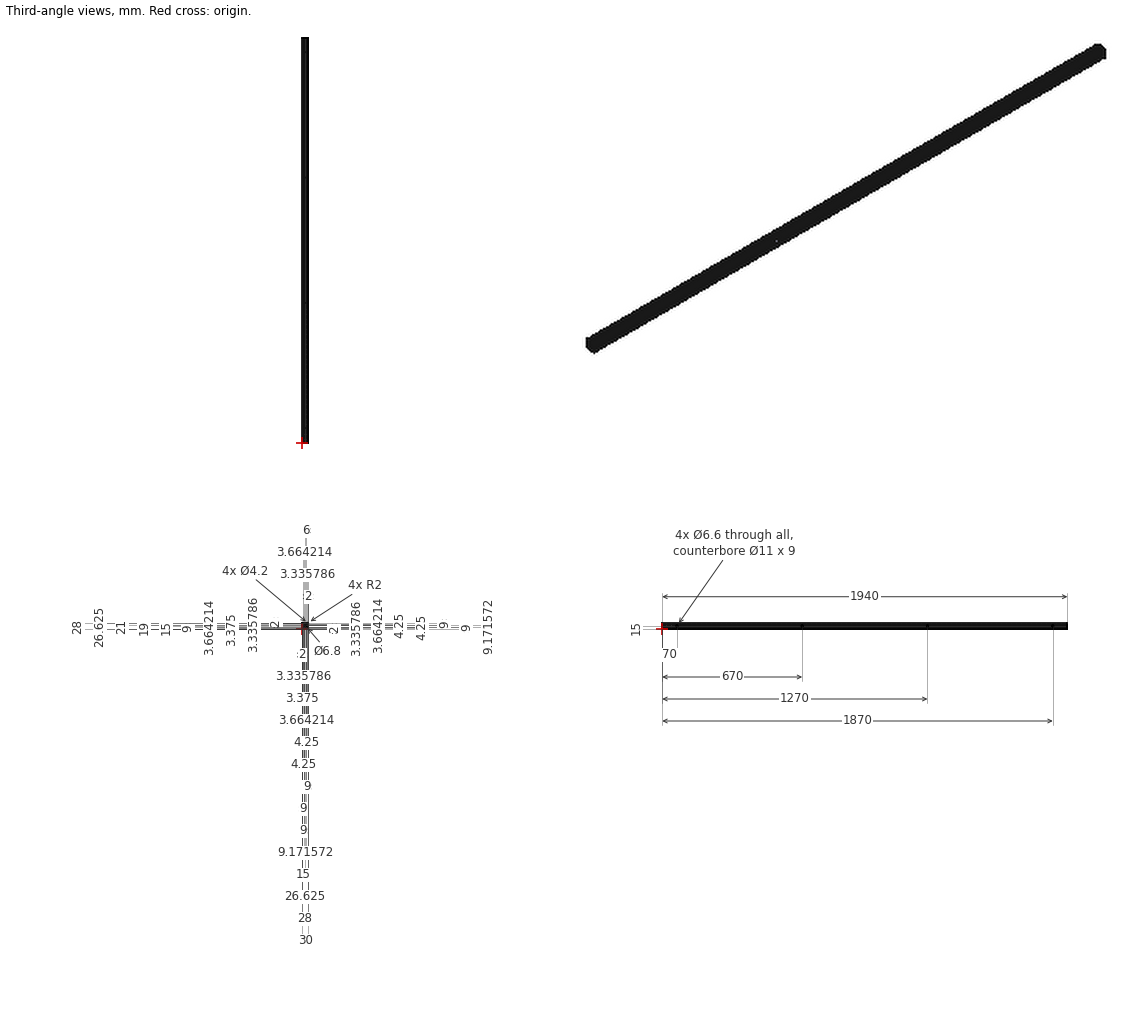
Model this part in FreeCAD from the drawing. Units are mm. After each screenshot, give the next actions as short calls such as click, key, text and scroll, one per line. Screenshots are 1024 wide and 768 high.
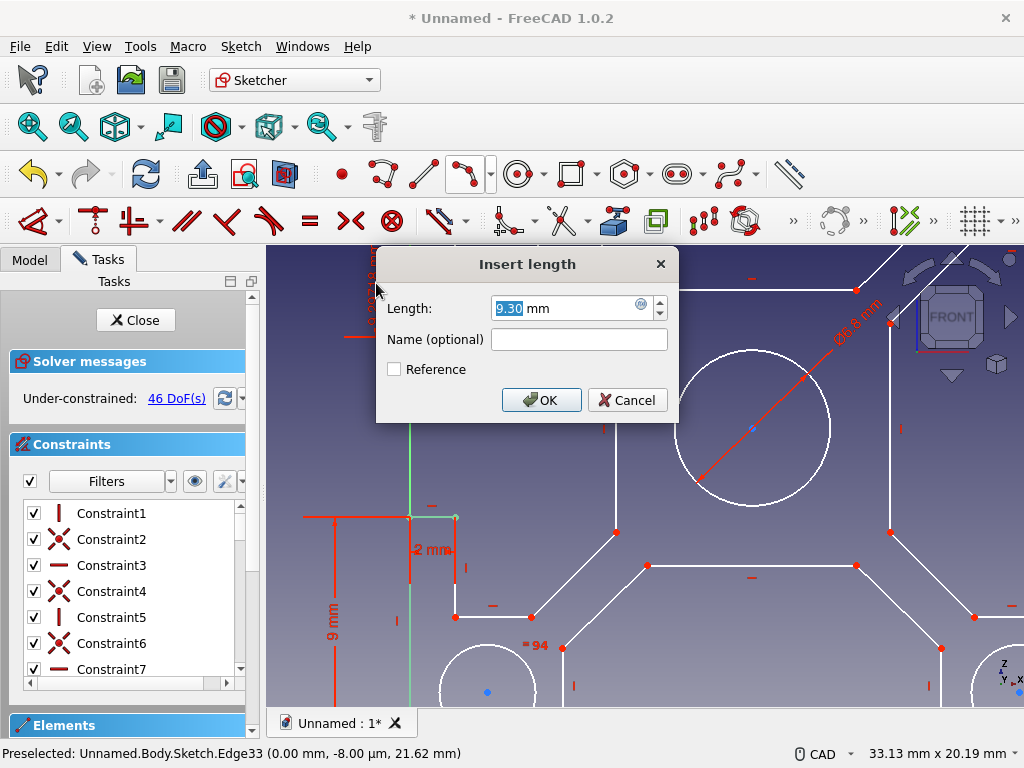
text(9)
key(Return)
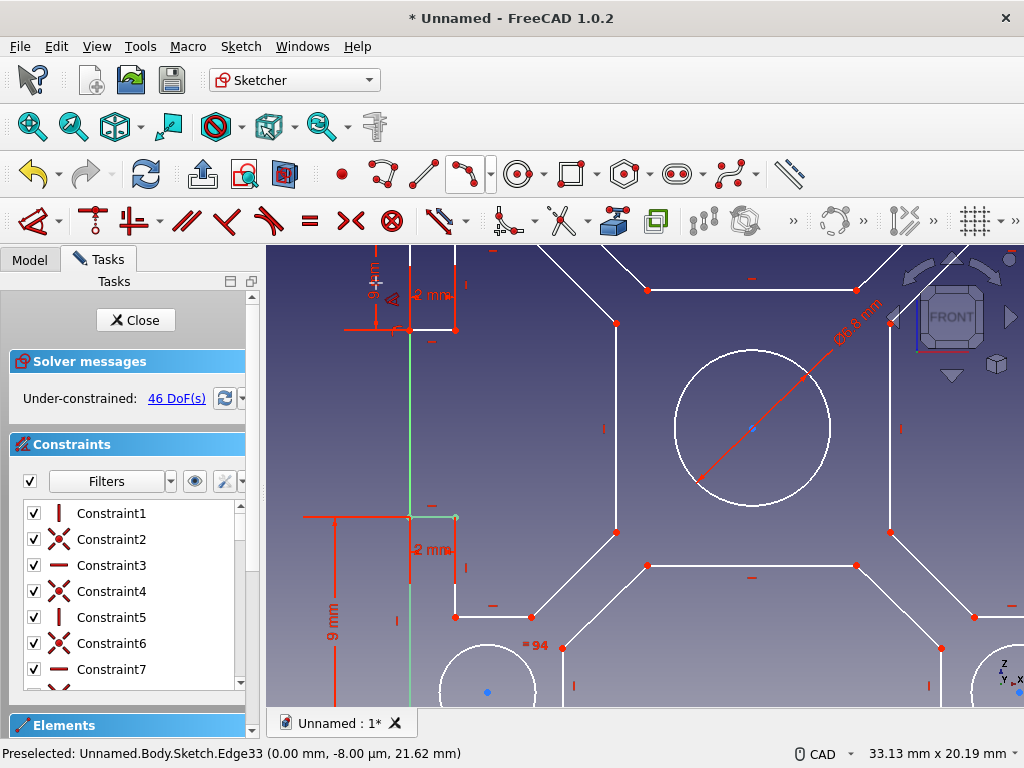
scroll(433, 517, down, 4)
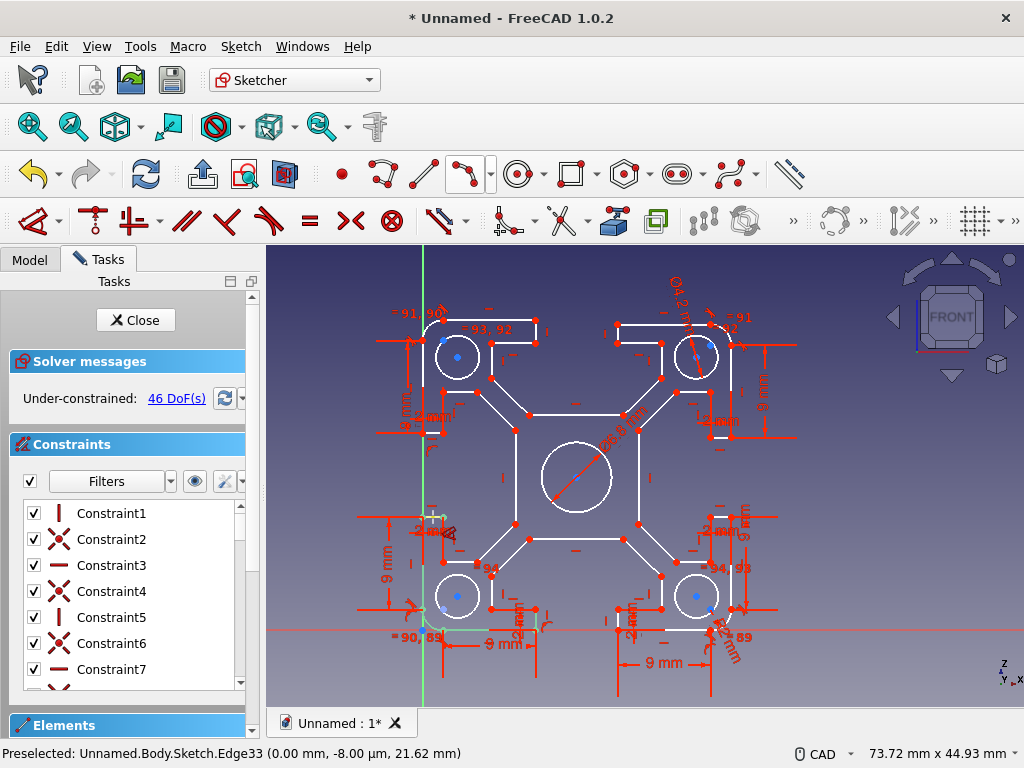
click(471, 320)
click(489, 286)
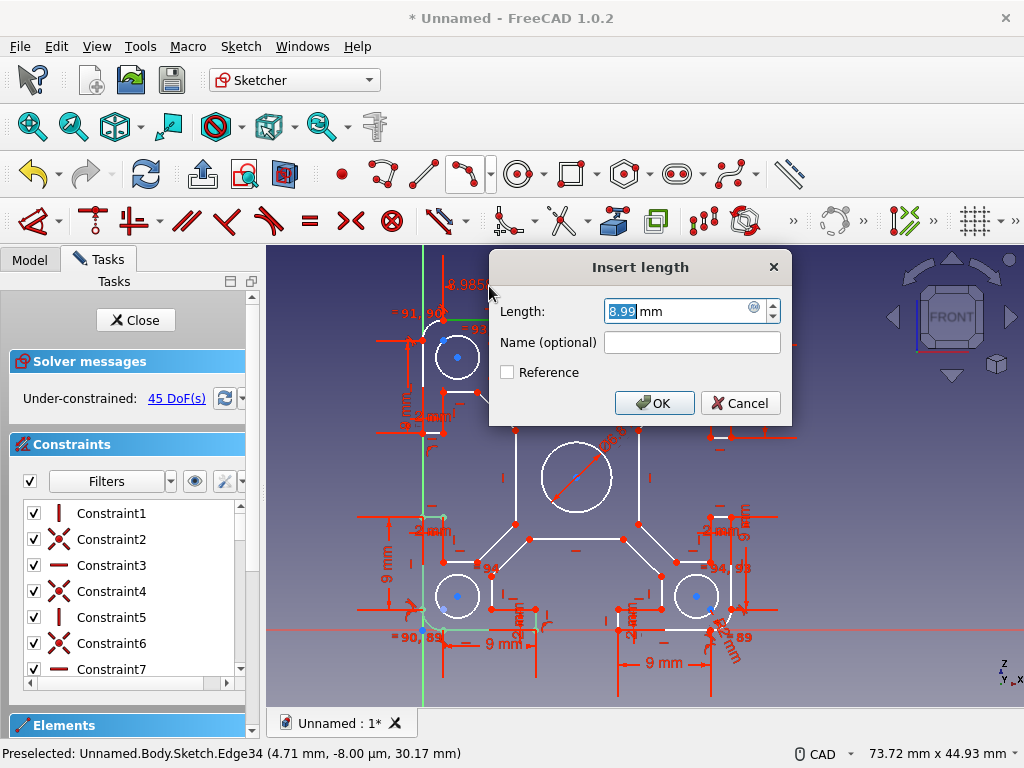
text(9)
key(Return)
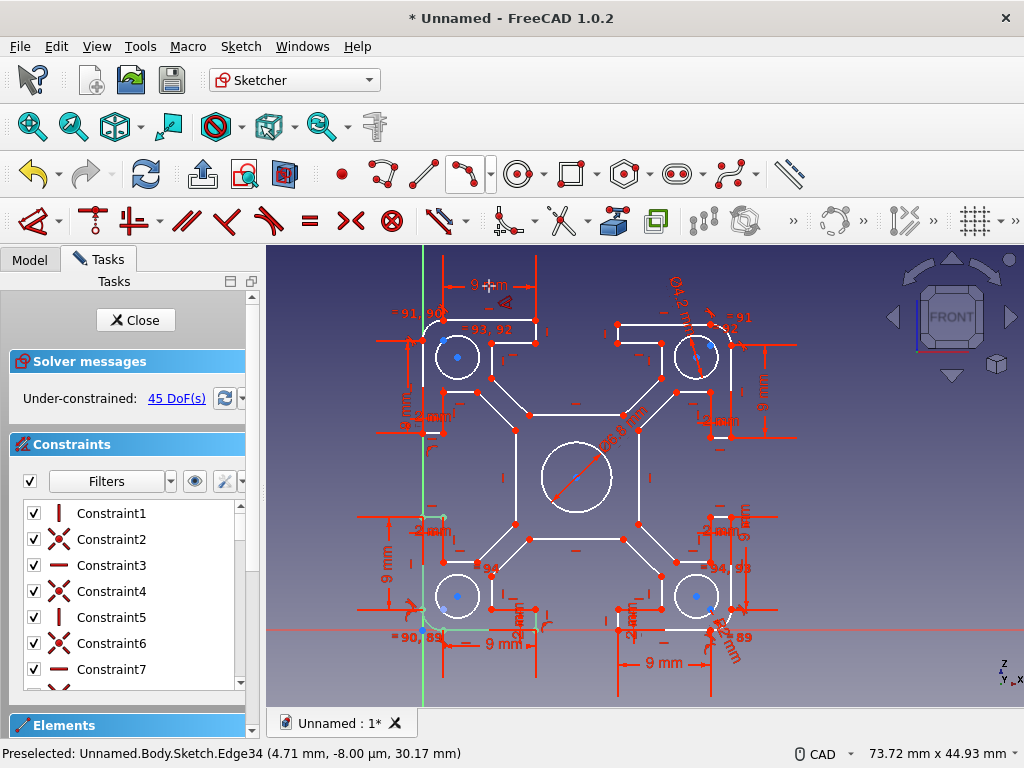
scroll(536, 329, up, 4)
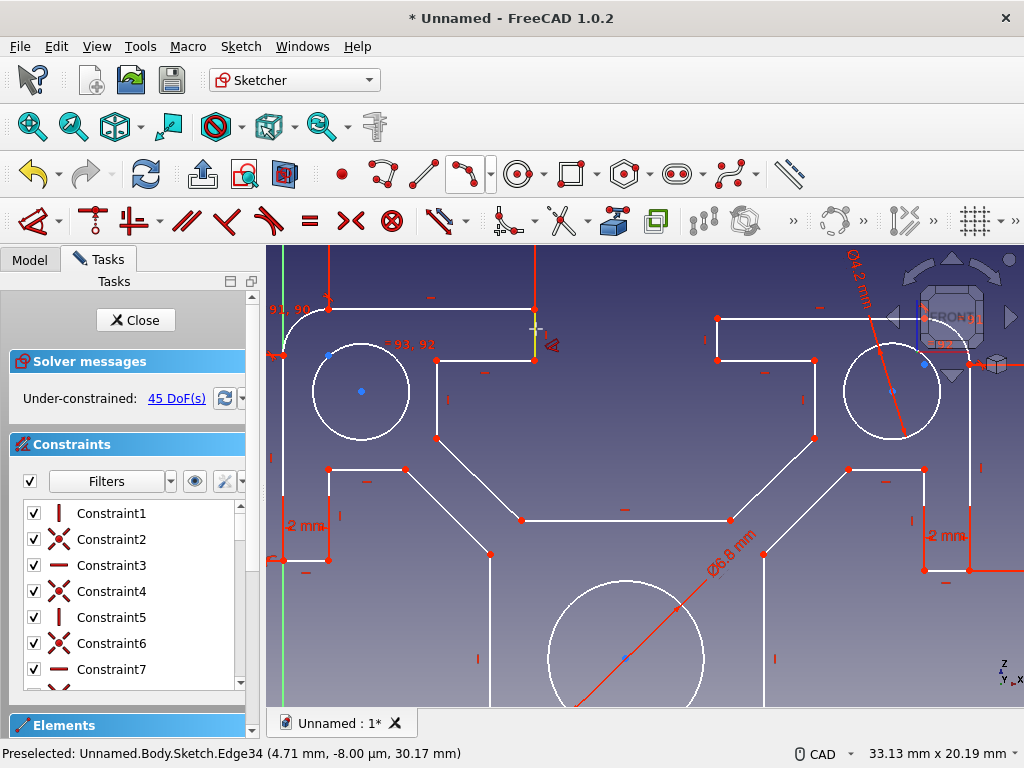
click(535, 330)
click(501, 335)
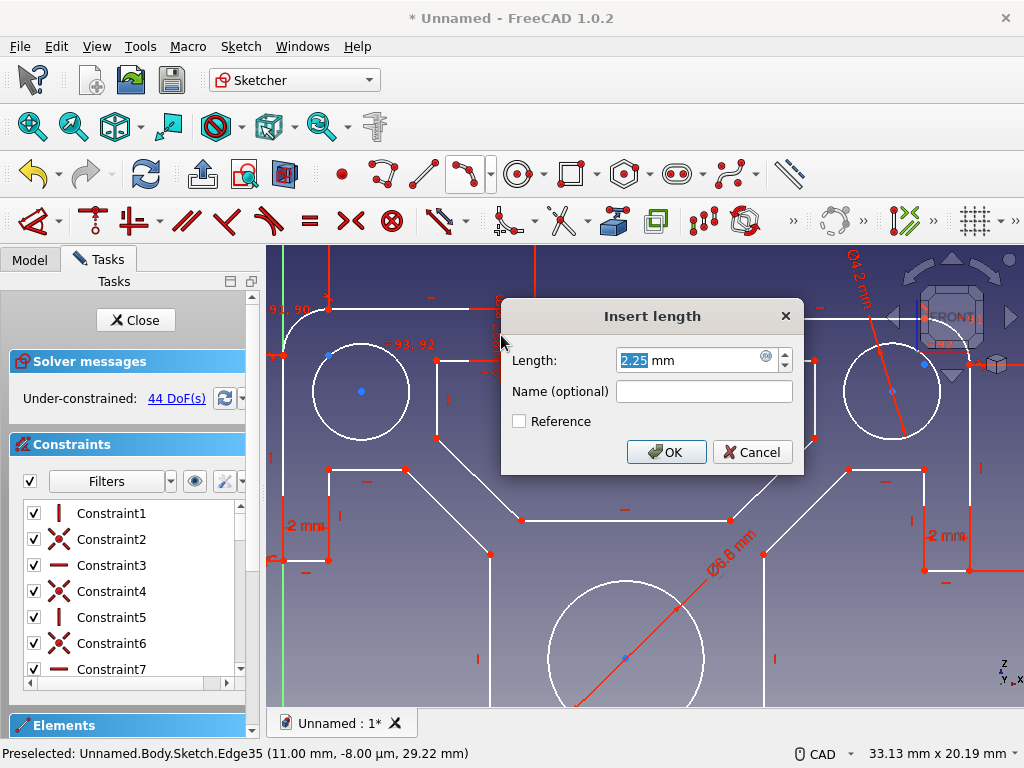
text(2)
key(Return)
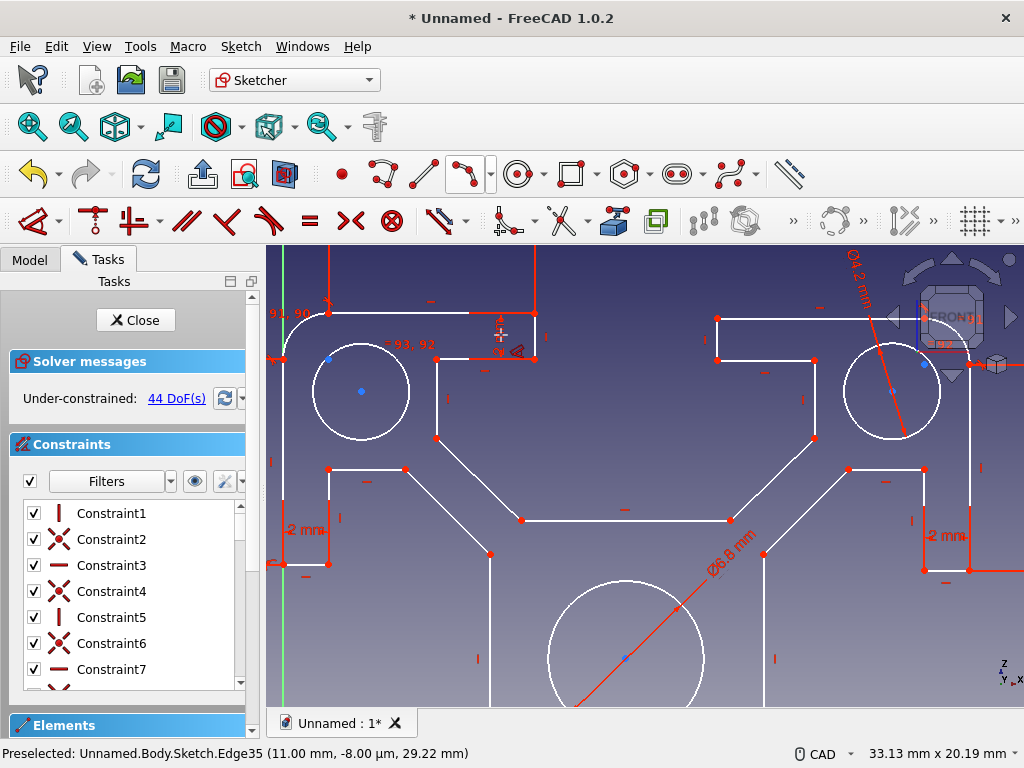
click(717, 348)
click(751, 340)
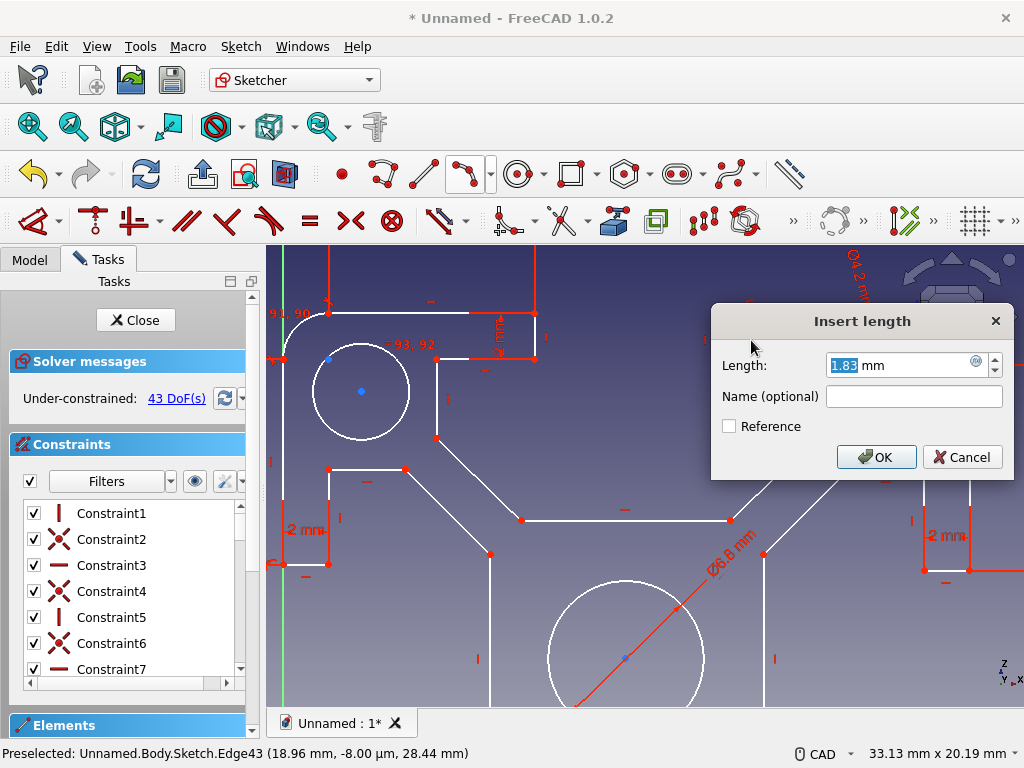
text(2)
key(Return)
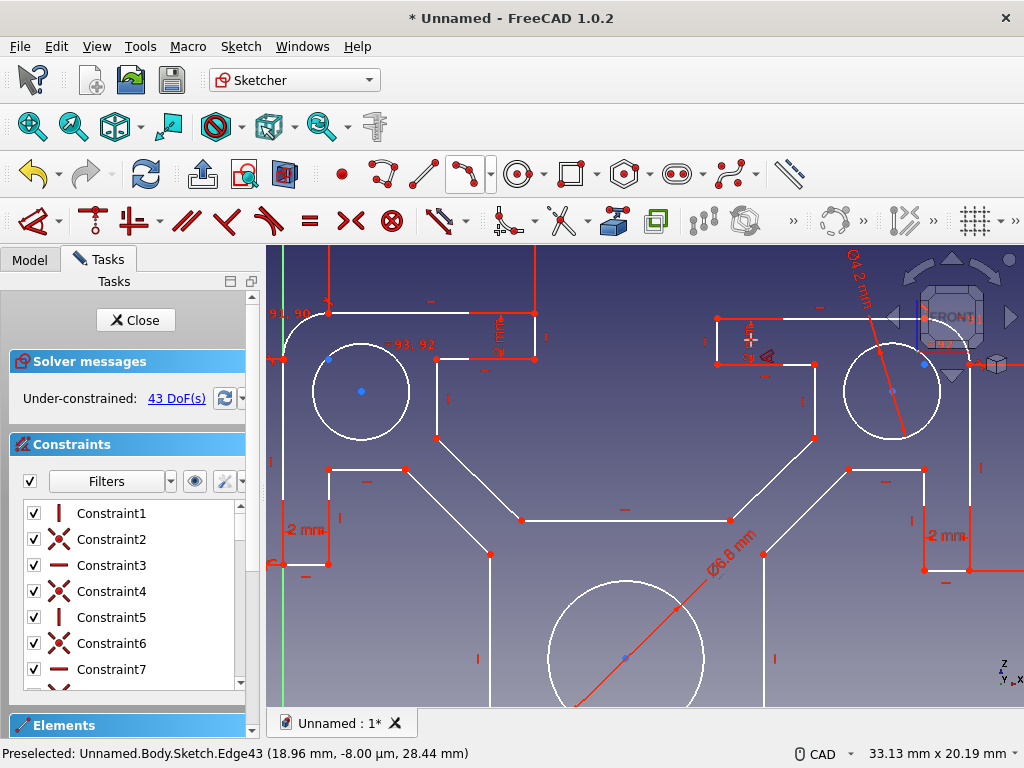
click(779, 319)
click(788, 285)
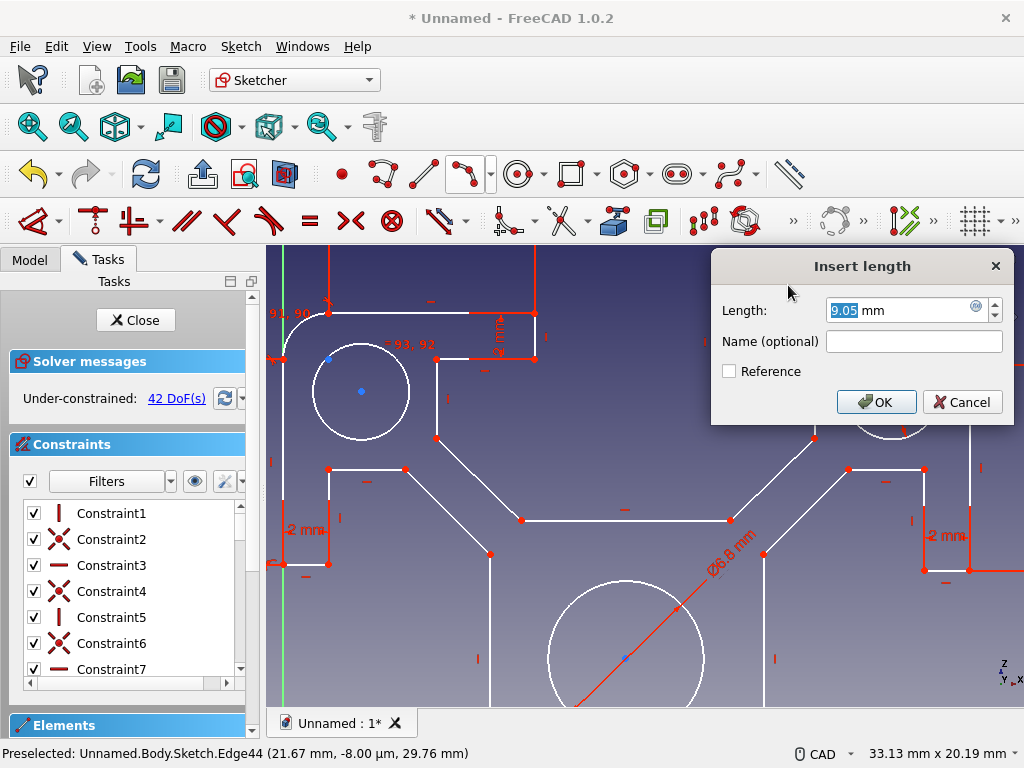
text(9)
key(Return)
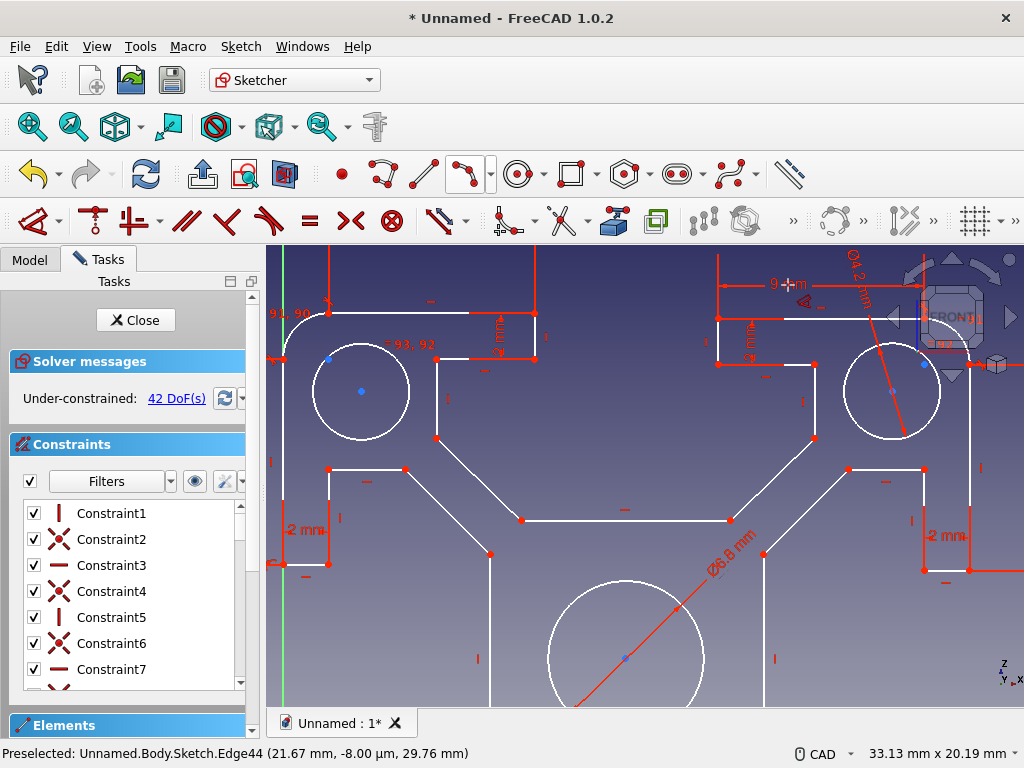
scroll(536, 329, down, 4)